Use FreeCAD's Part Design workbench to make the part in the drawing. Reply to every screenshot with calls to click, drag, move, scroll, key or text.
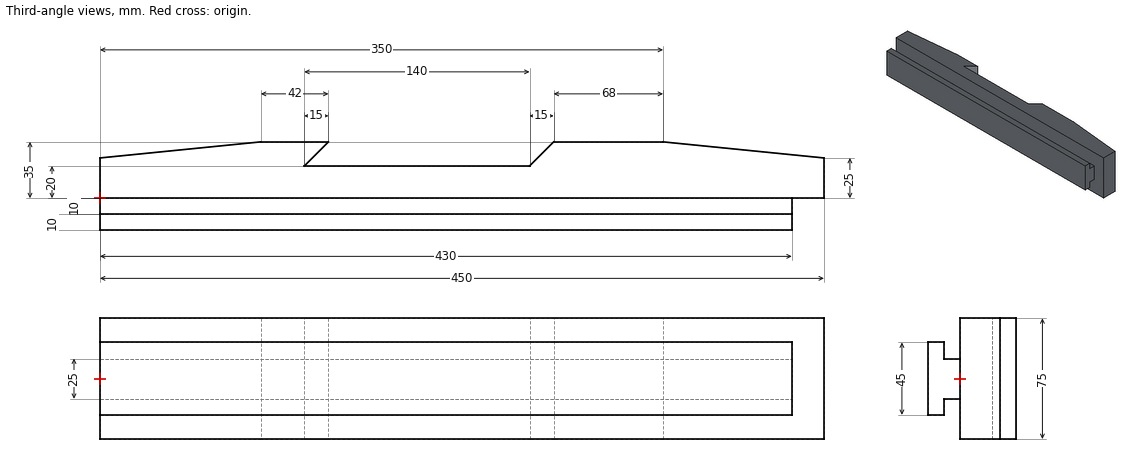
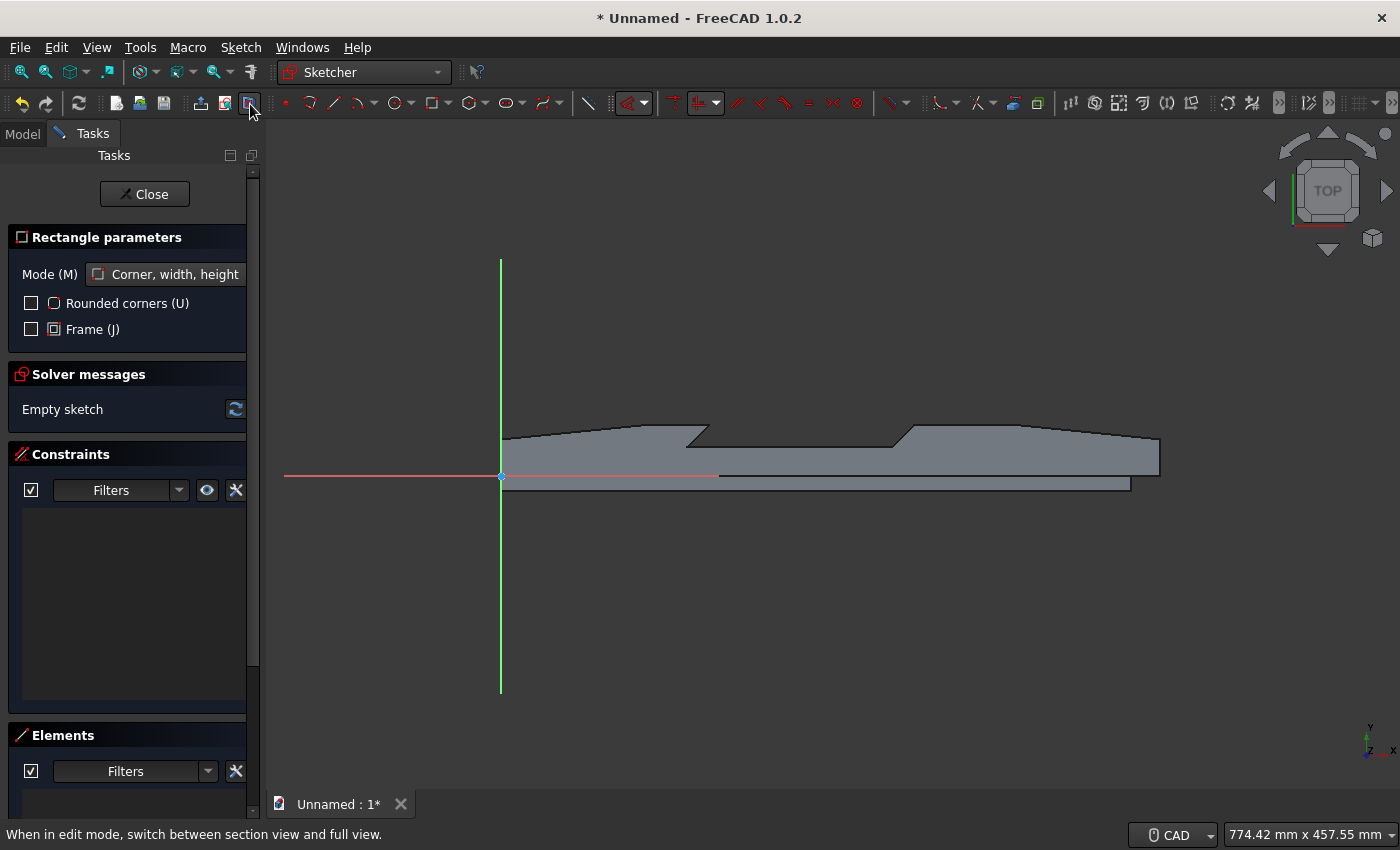
click(501, 491)
click(1131, 505)
key(Escape)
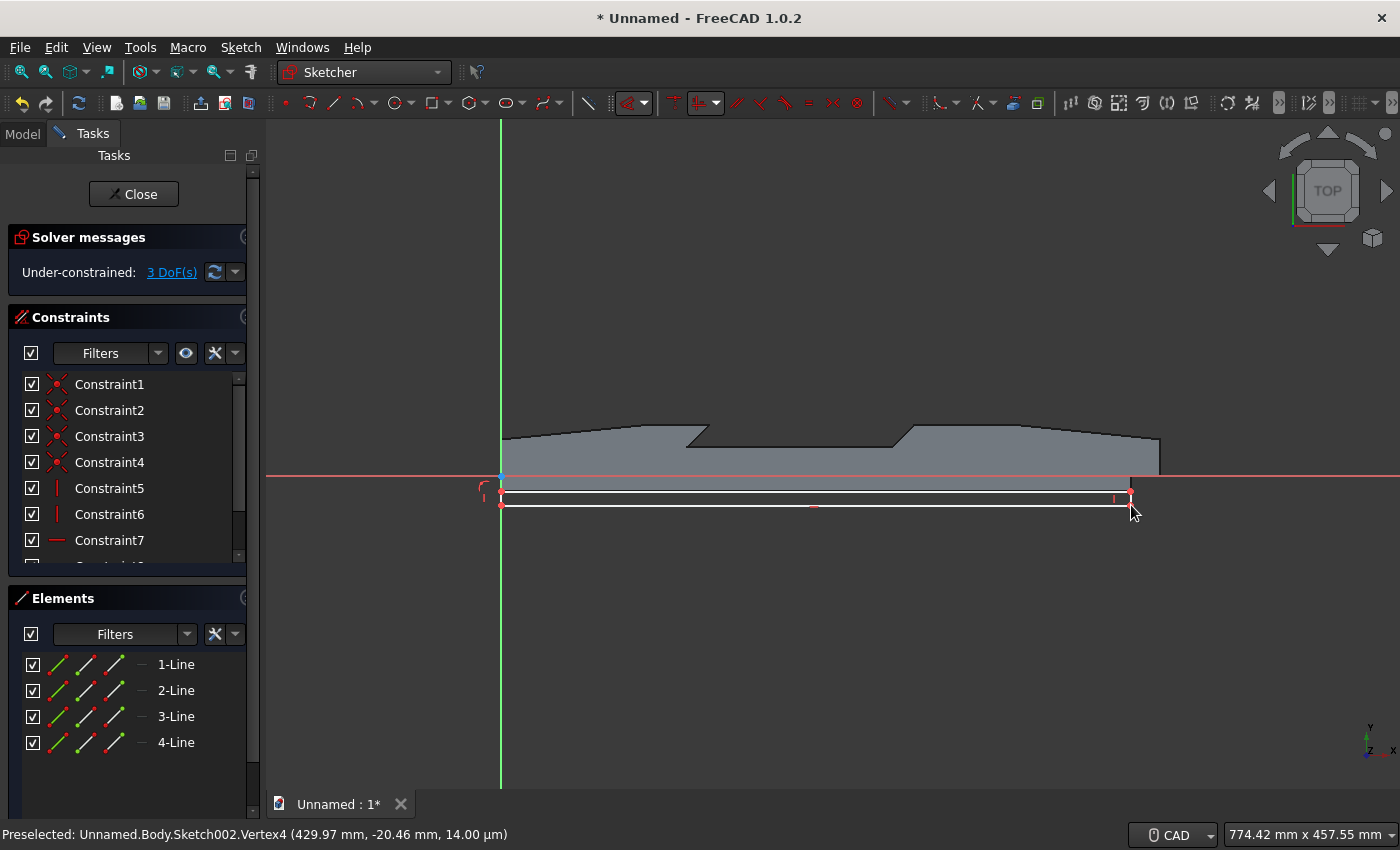
scroll(501, 499, up, 5)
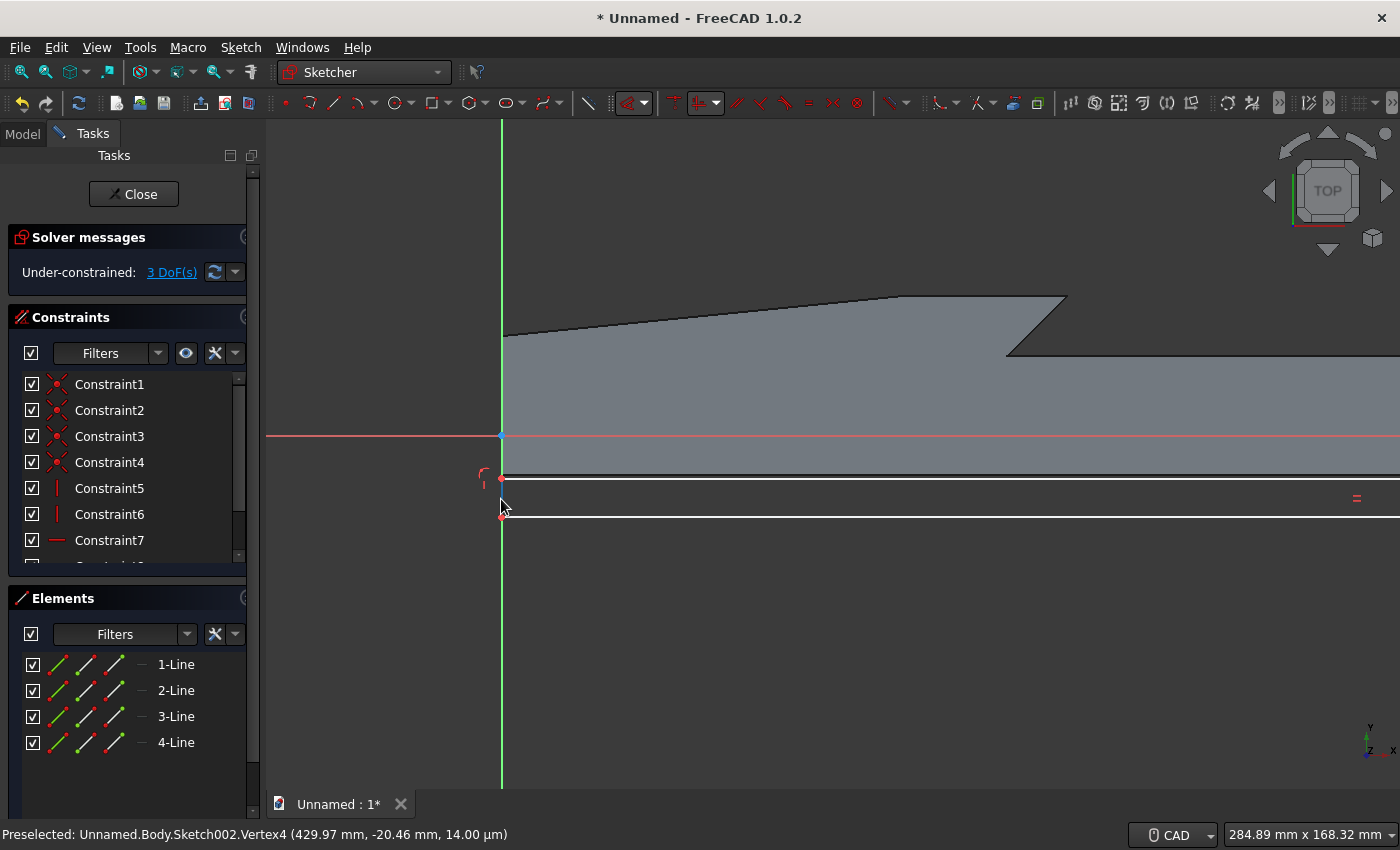
click(502, 498)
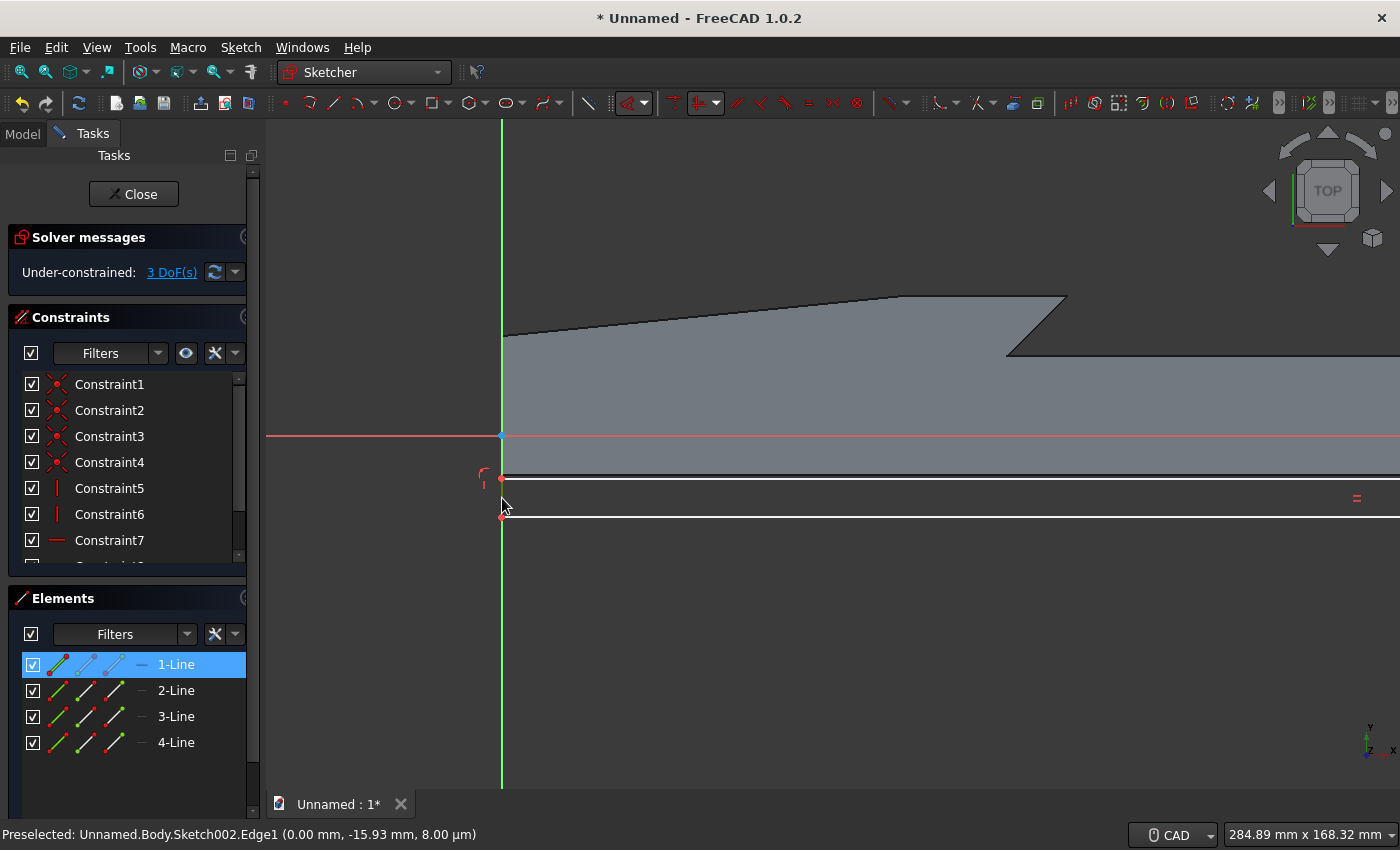
key(i)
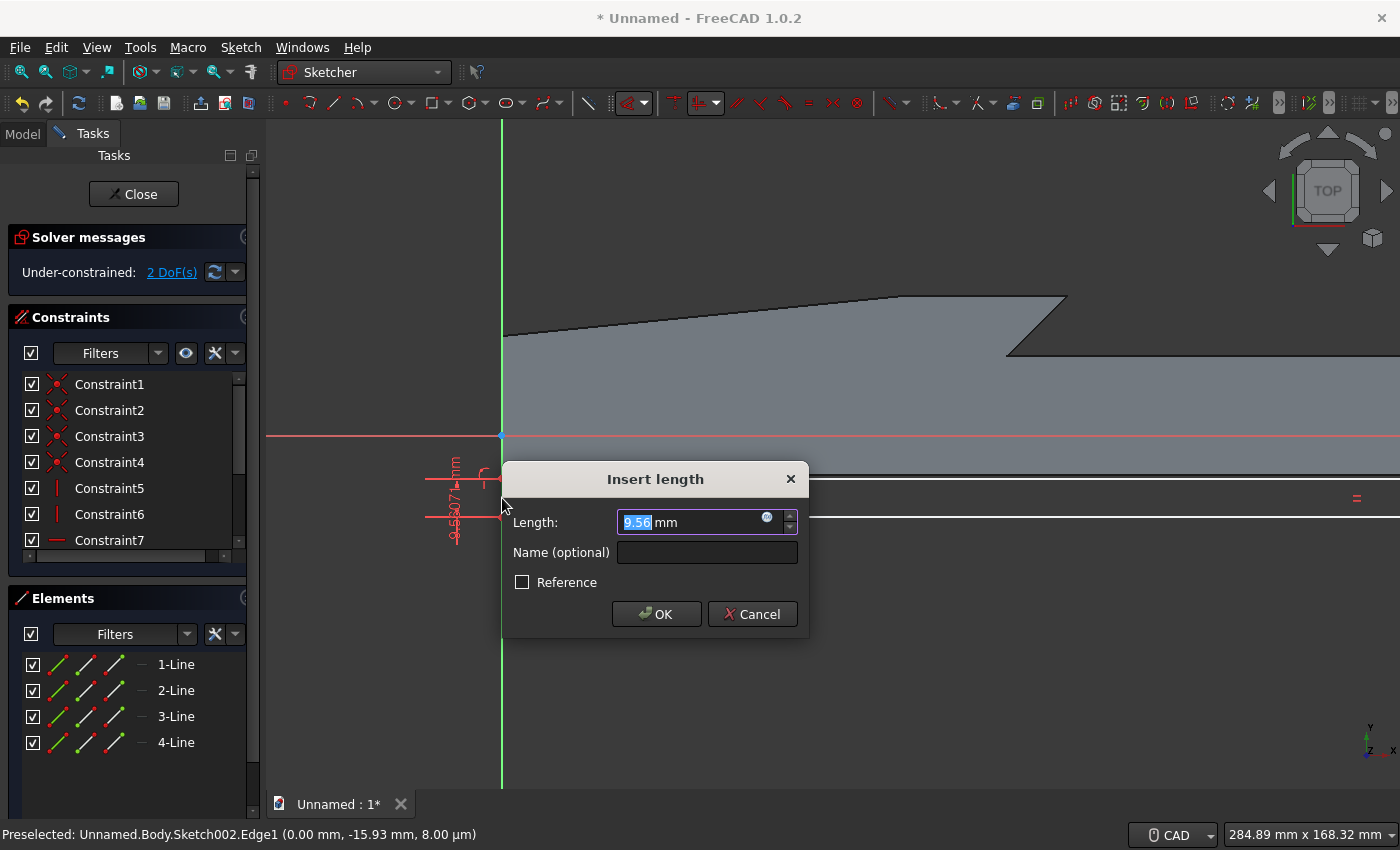
text(10)
key(Return)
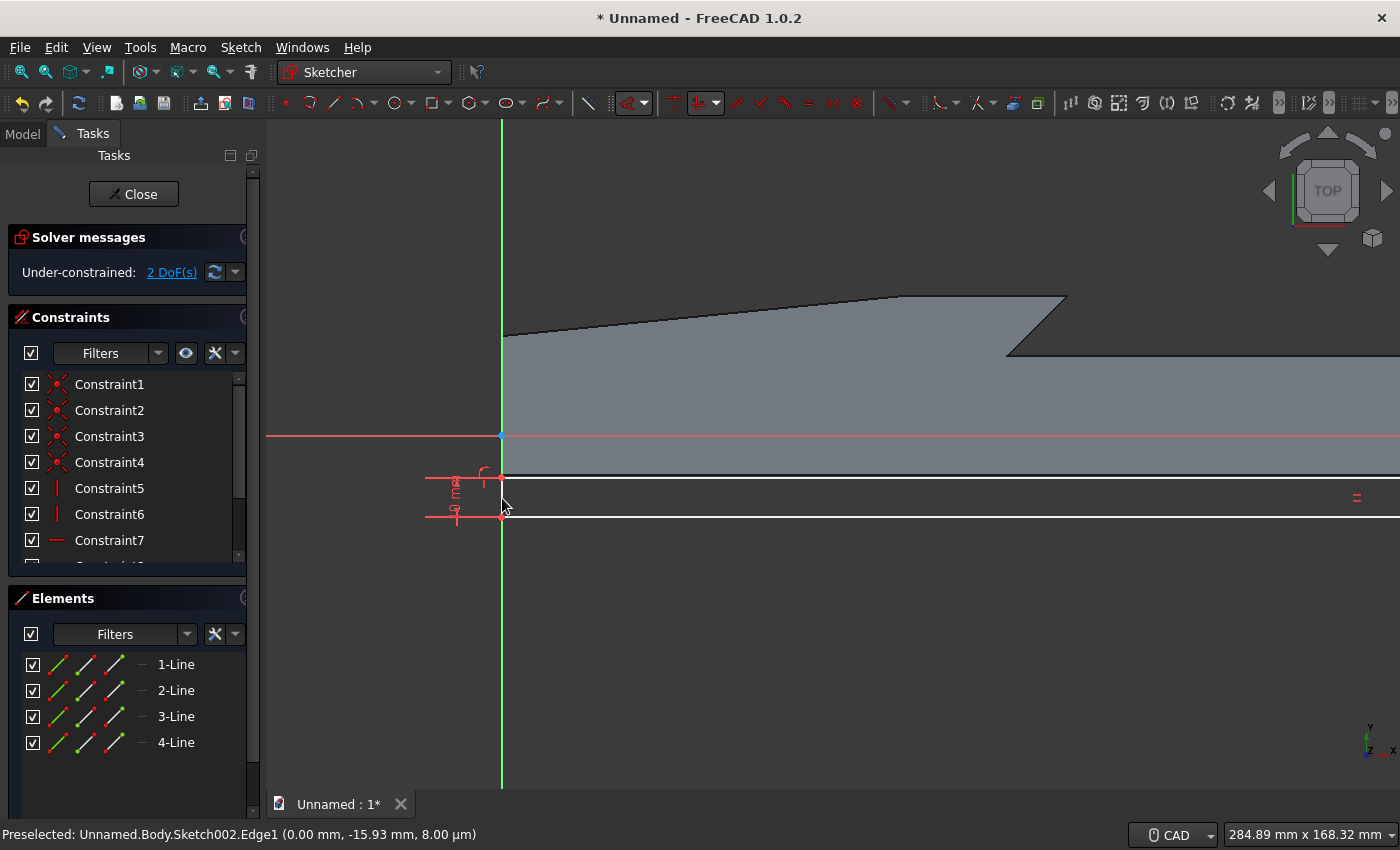
click(1015, 517)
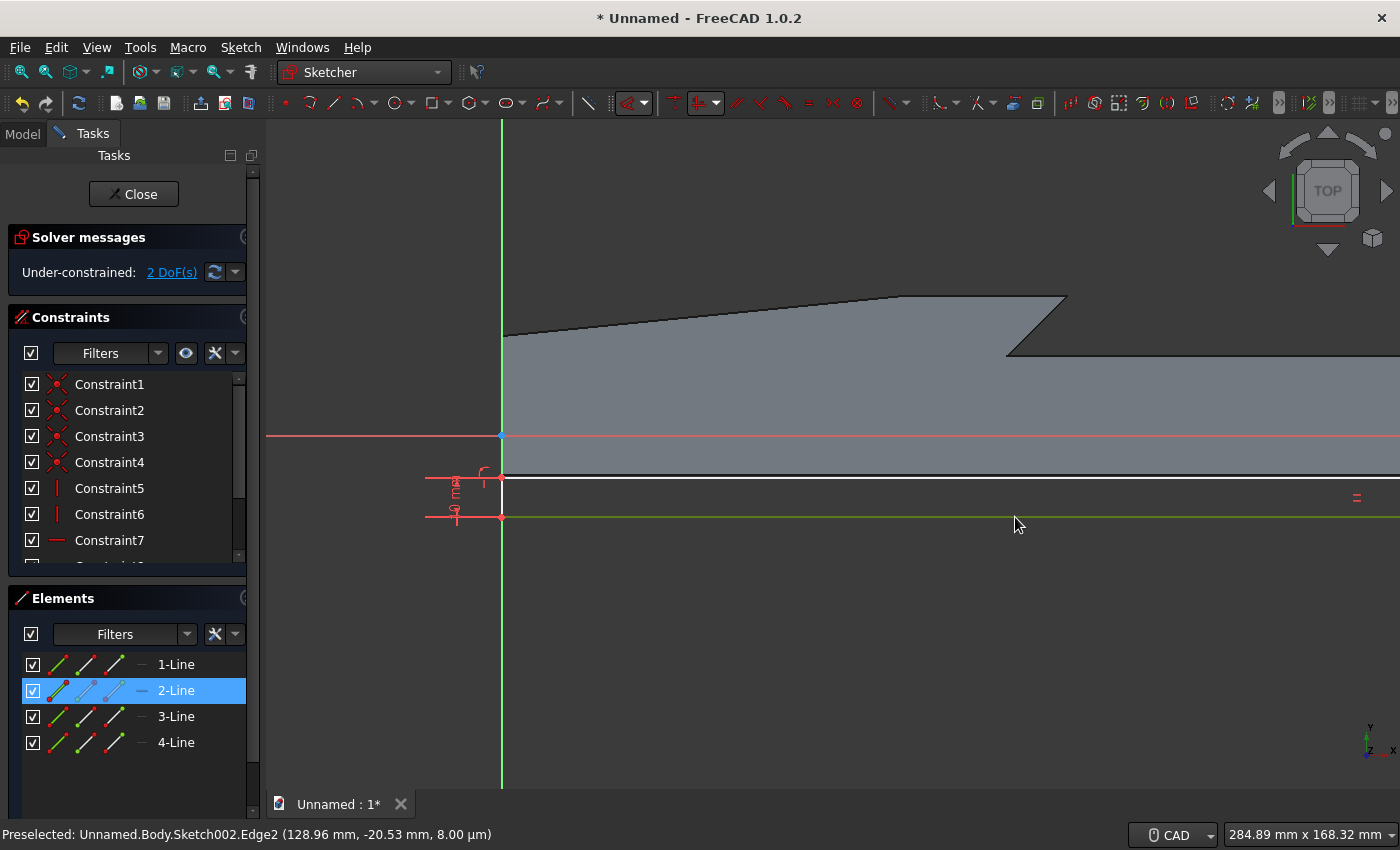
key(l)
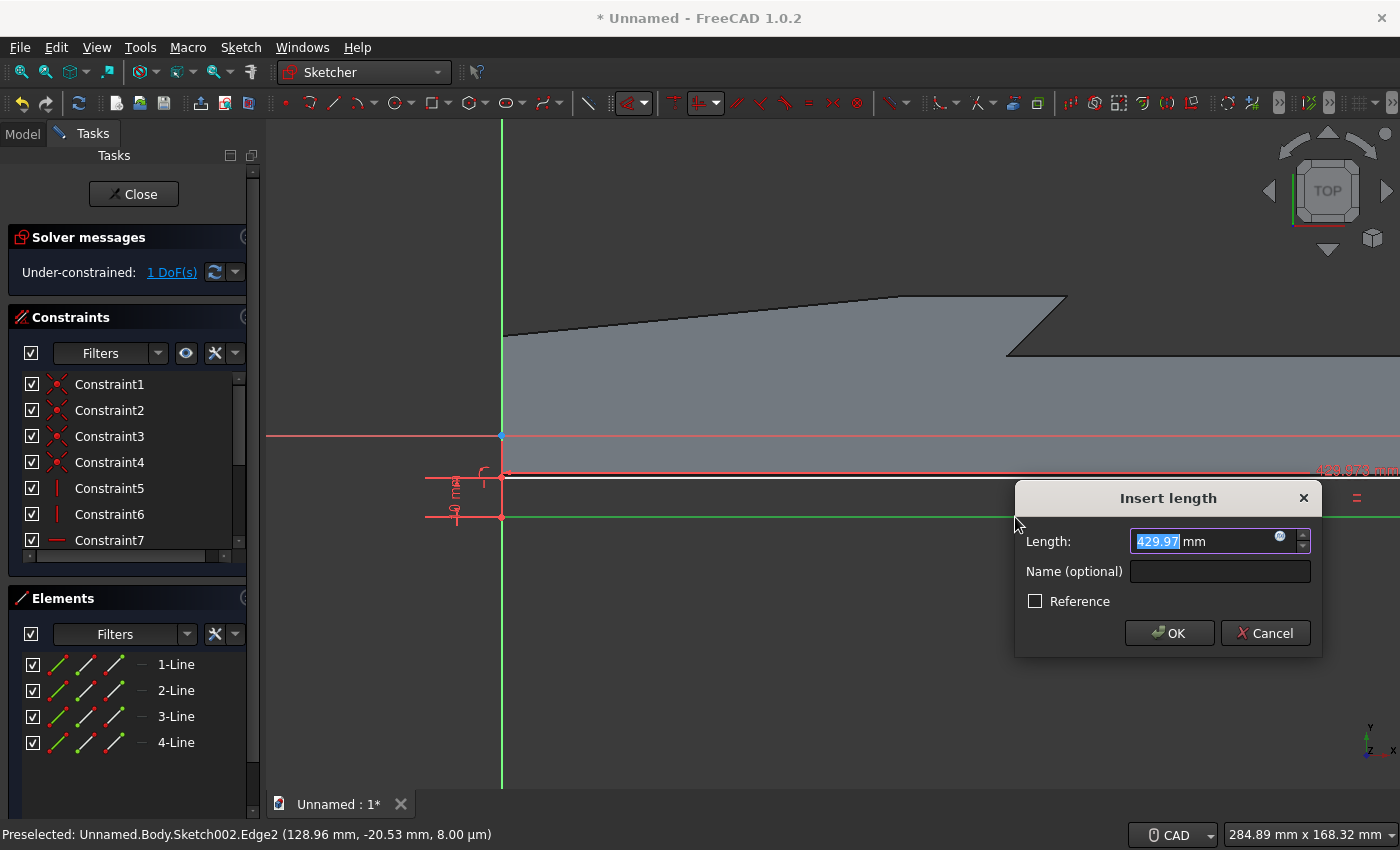
text(430)
key(Return)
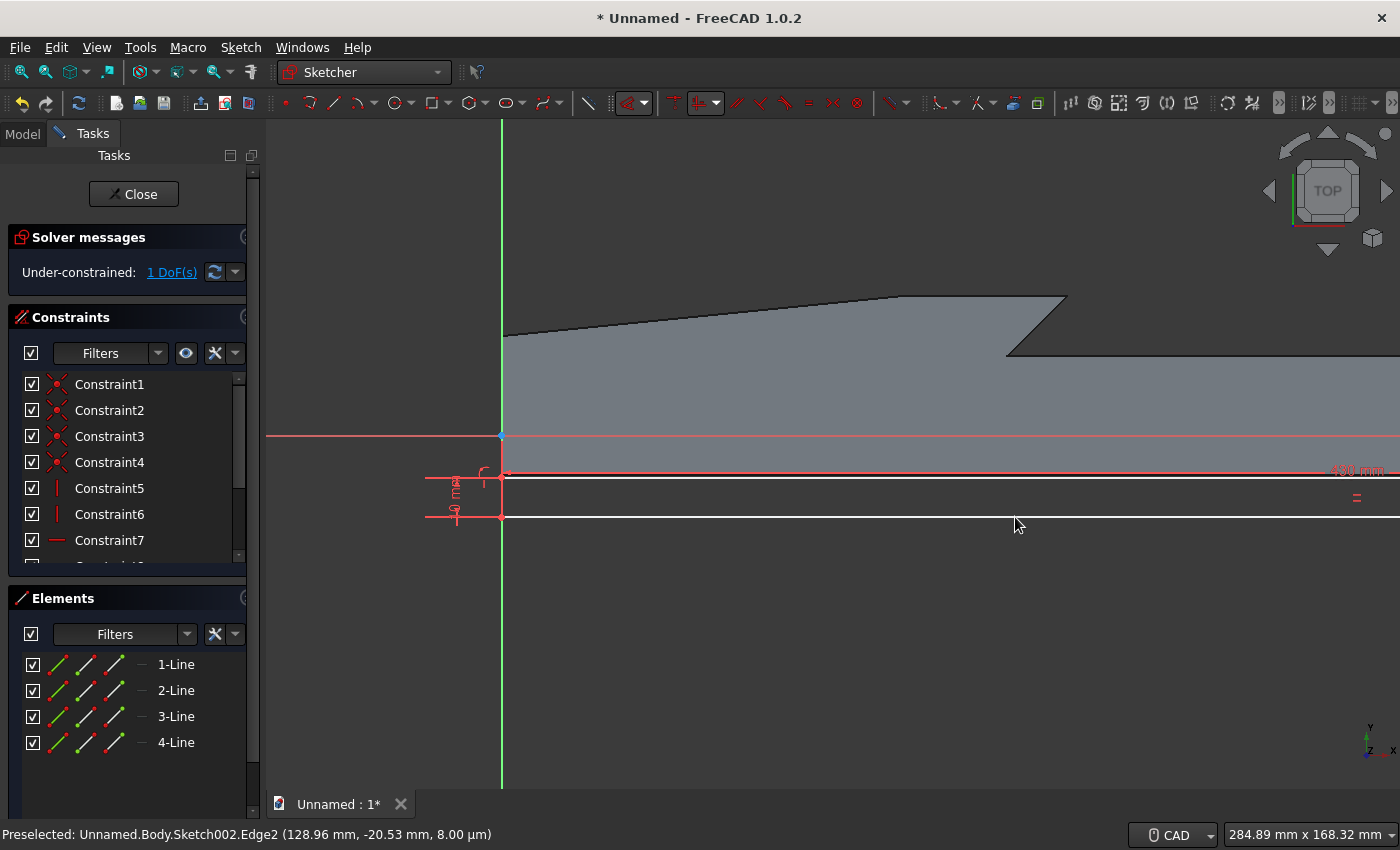
click(502, 478)